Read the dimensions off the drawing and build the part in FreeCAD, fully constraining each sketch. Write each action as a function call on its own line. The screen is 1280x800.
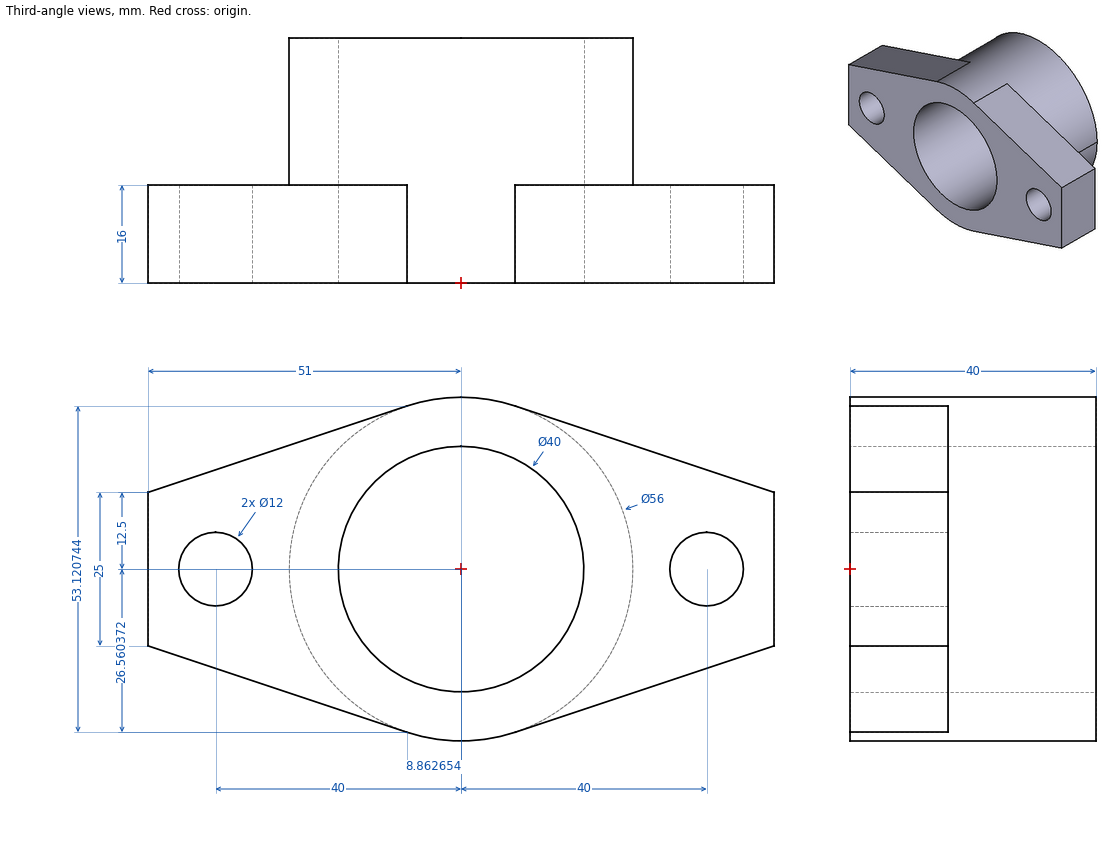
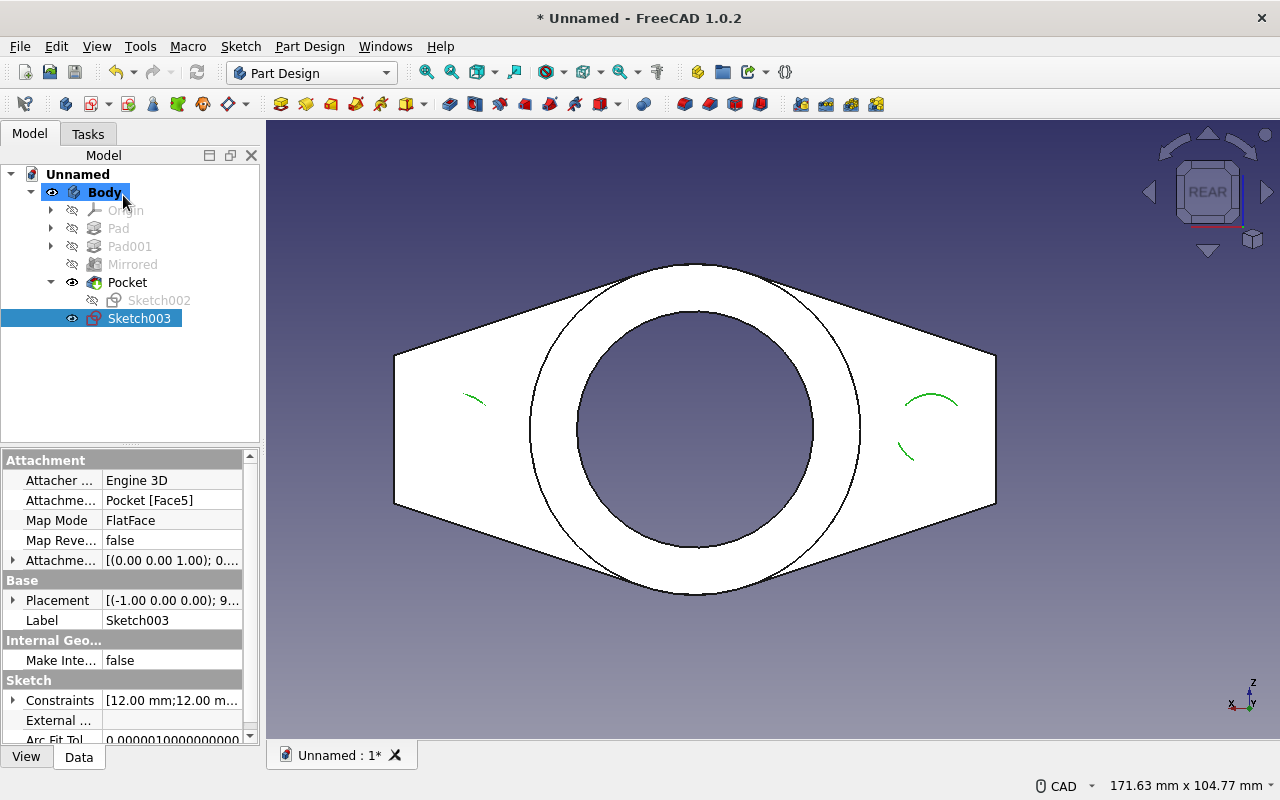
click(450, 104)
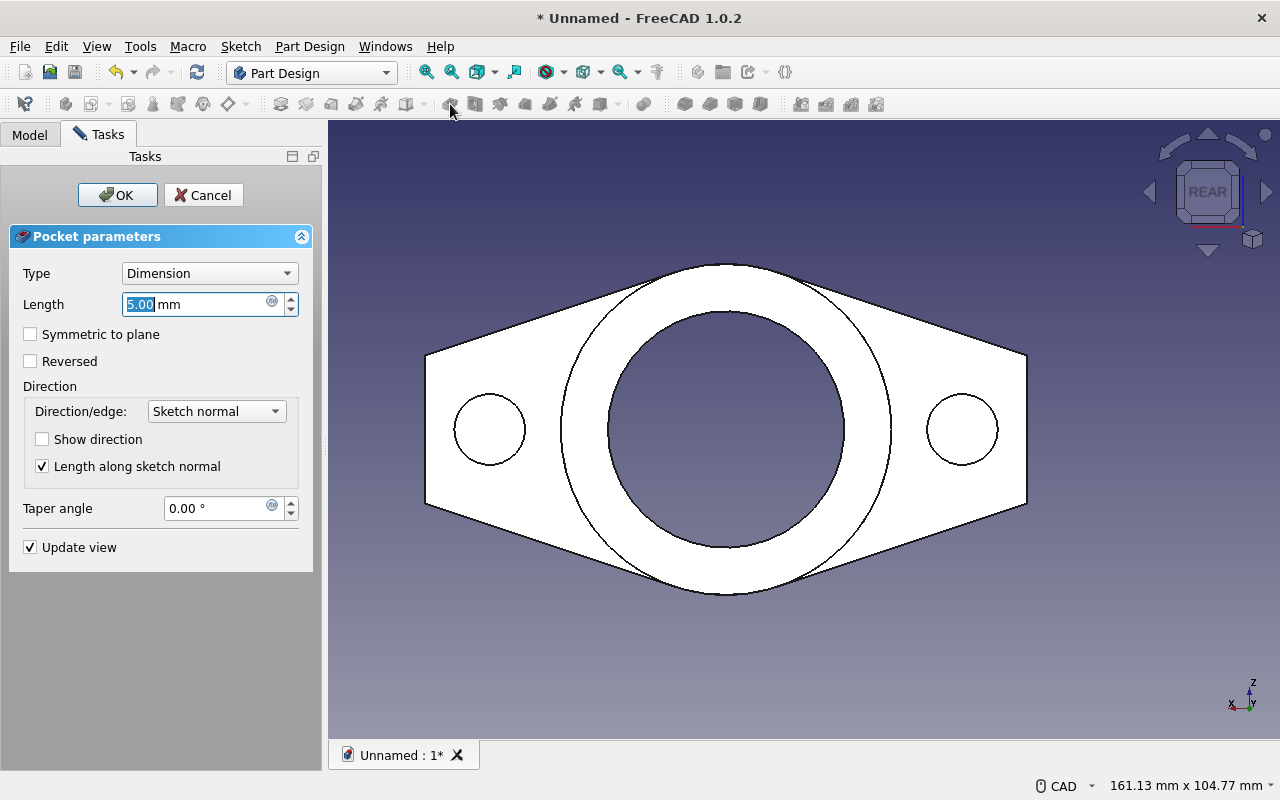
click(210, 274)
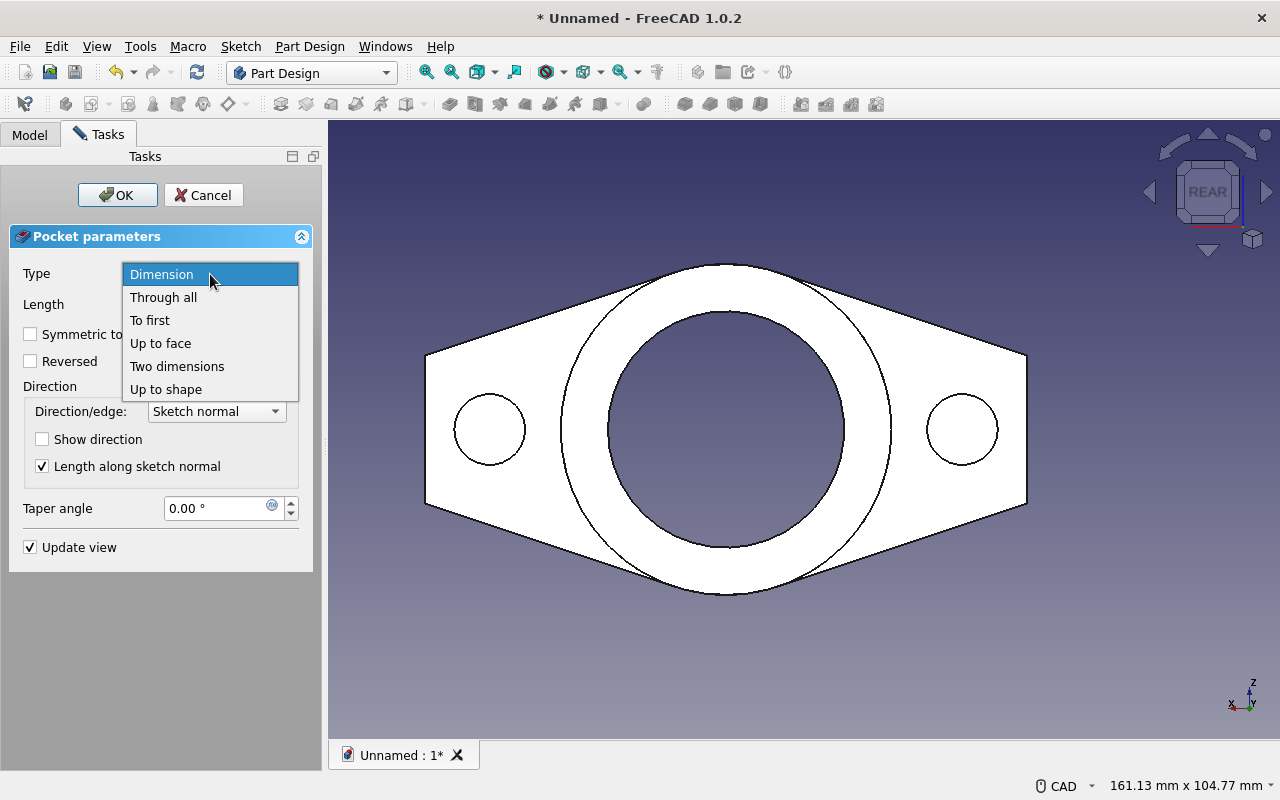
click(208, 298)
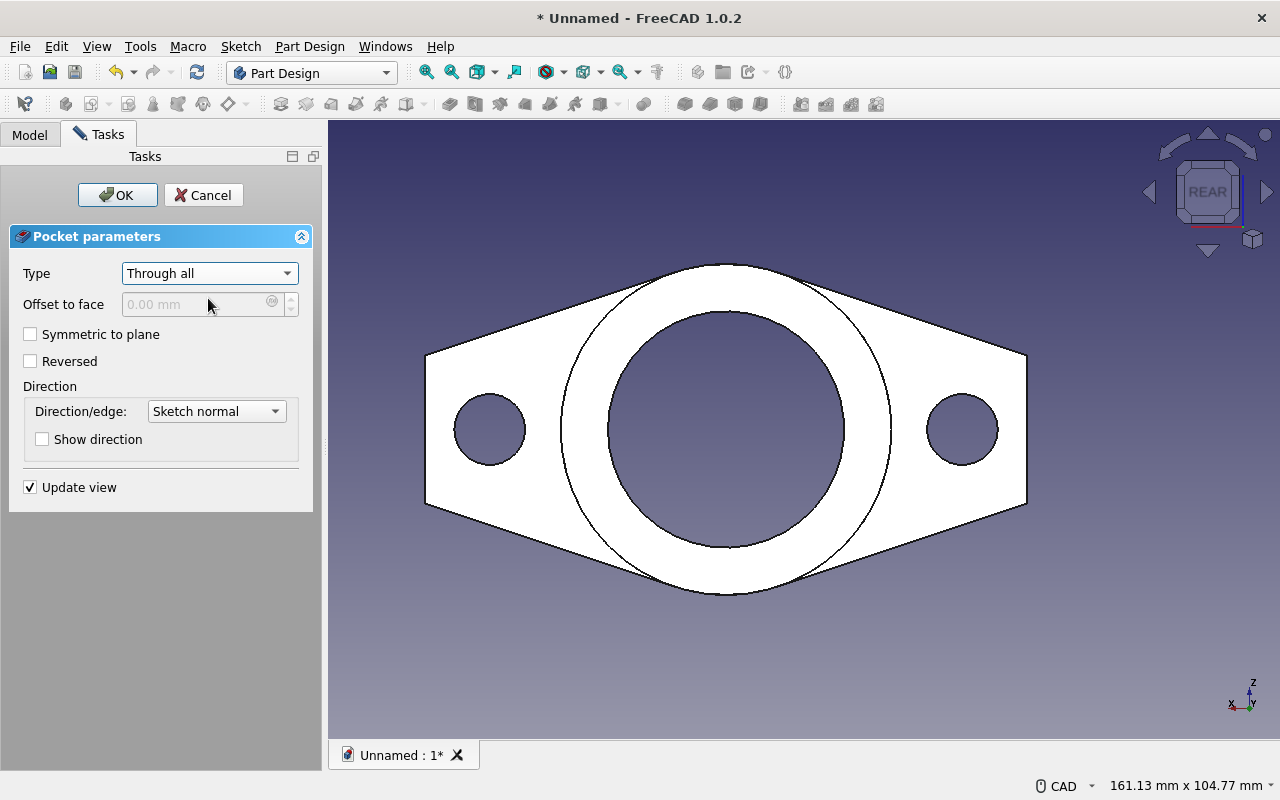
click(118, 195)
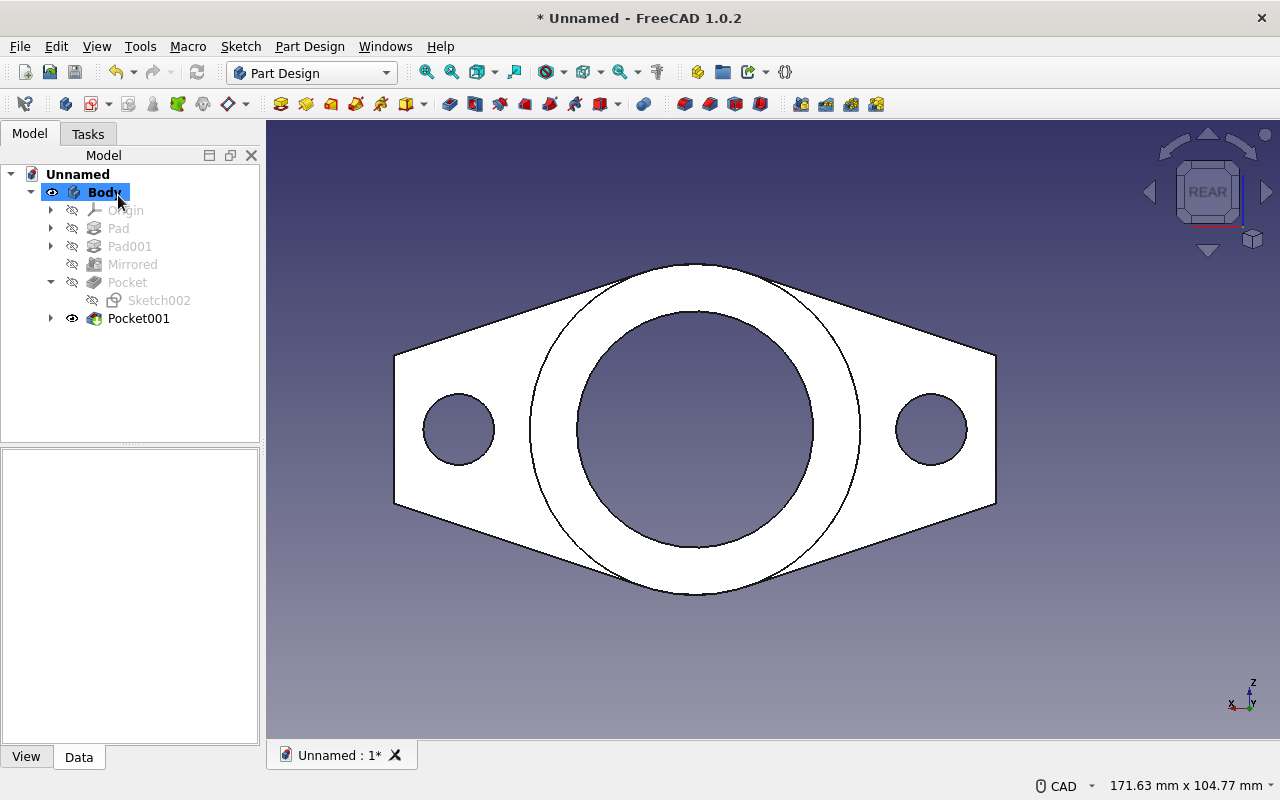
key(0)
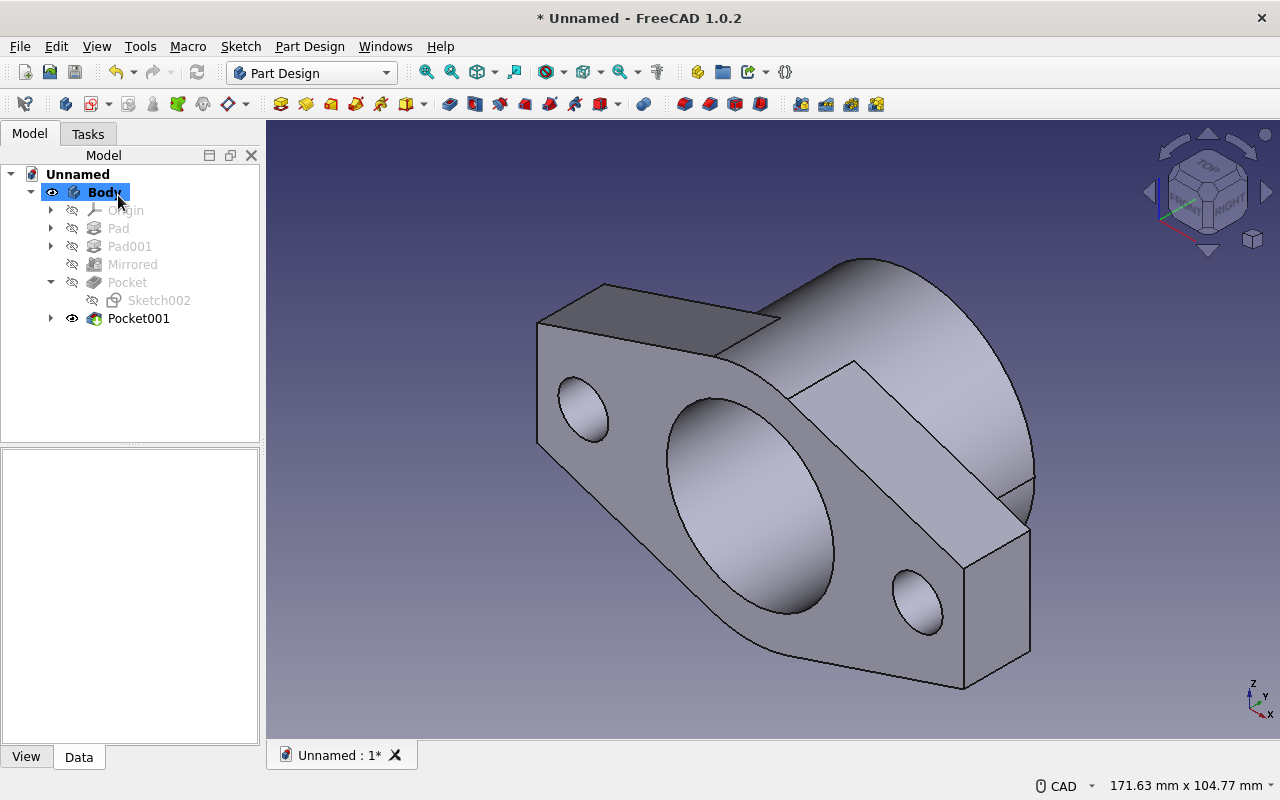
click(427, 72)